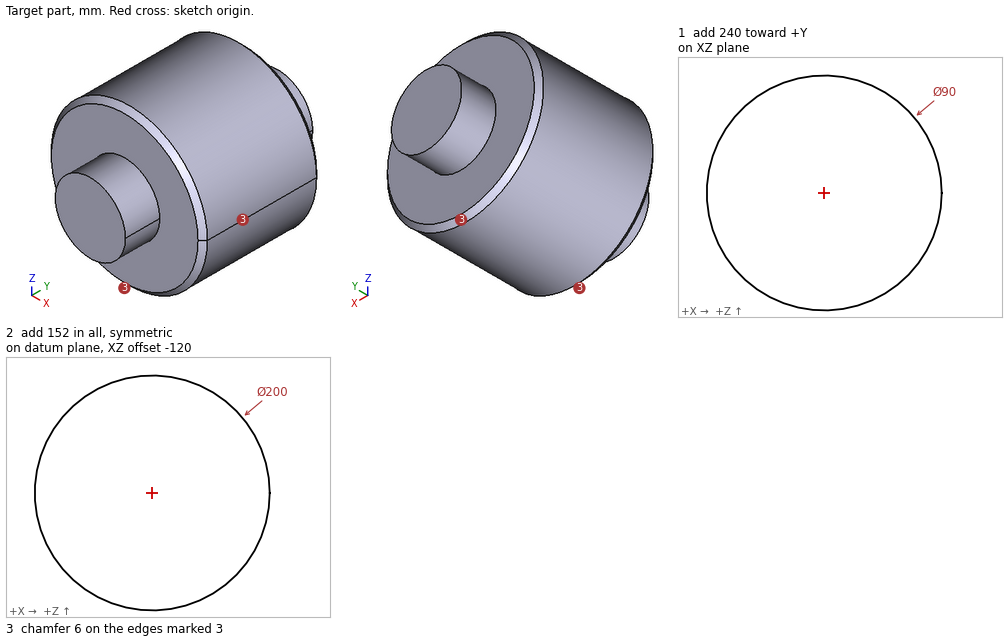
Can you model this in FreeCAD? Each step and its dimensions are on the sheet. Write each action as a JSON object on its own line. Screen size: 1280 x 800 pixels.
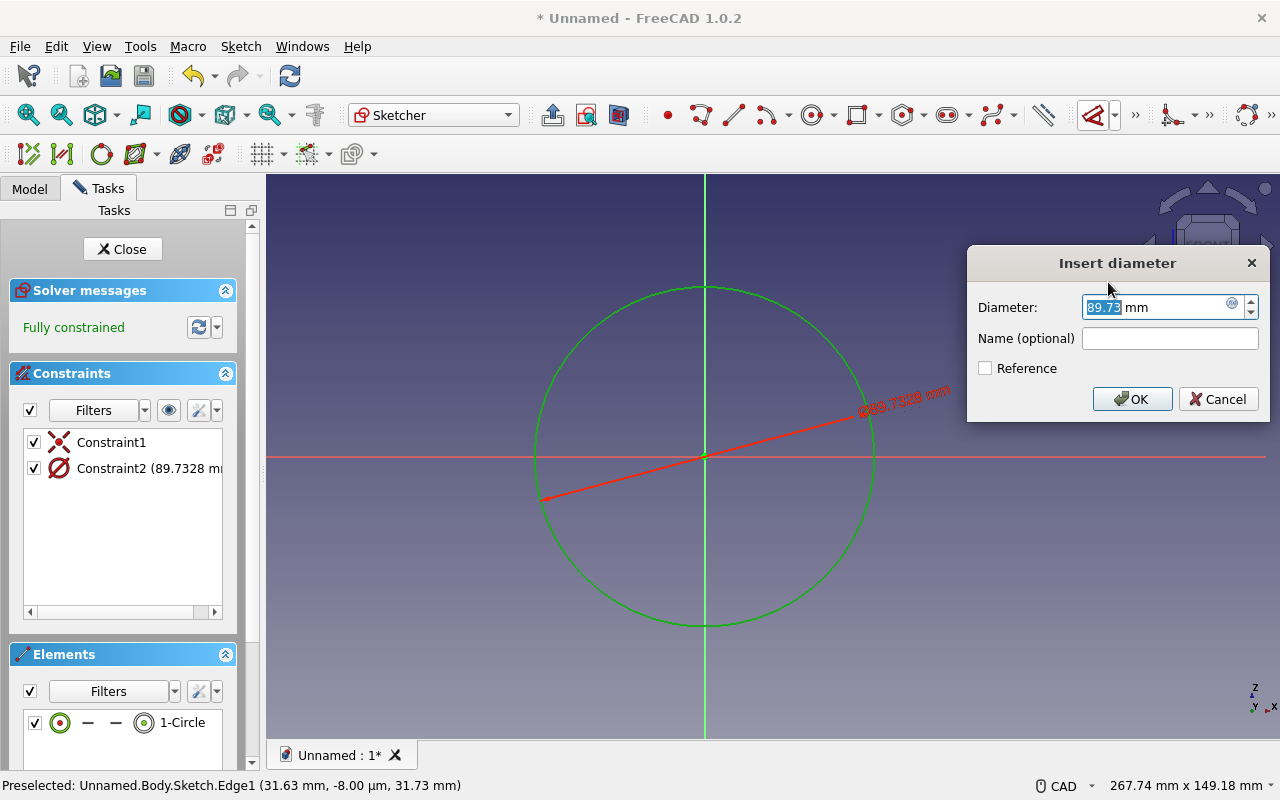
{"action": "type", "text": "90"}
{"action": "key", "text": "Return"}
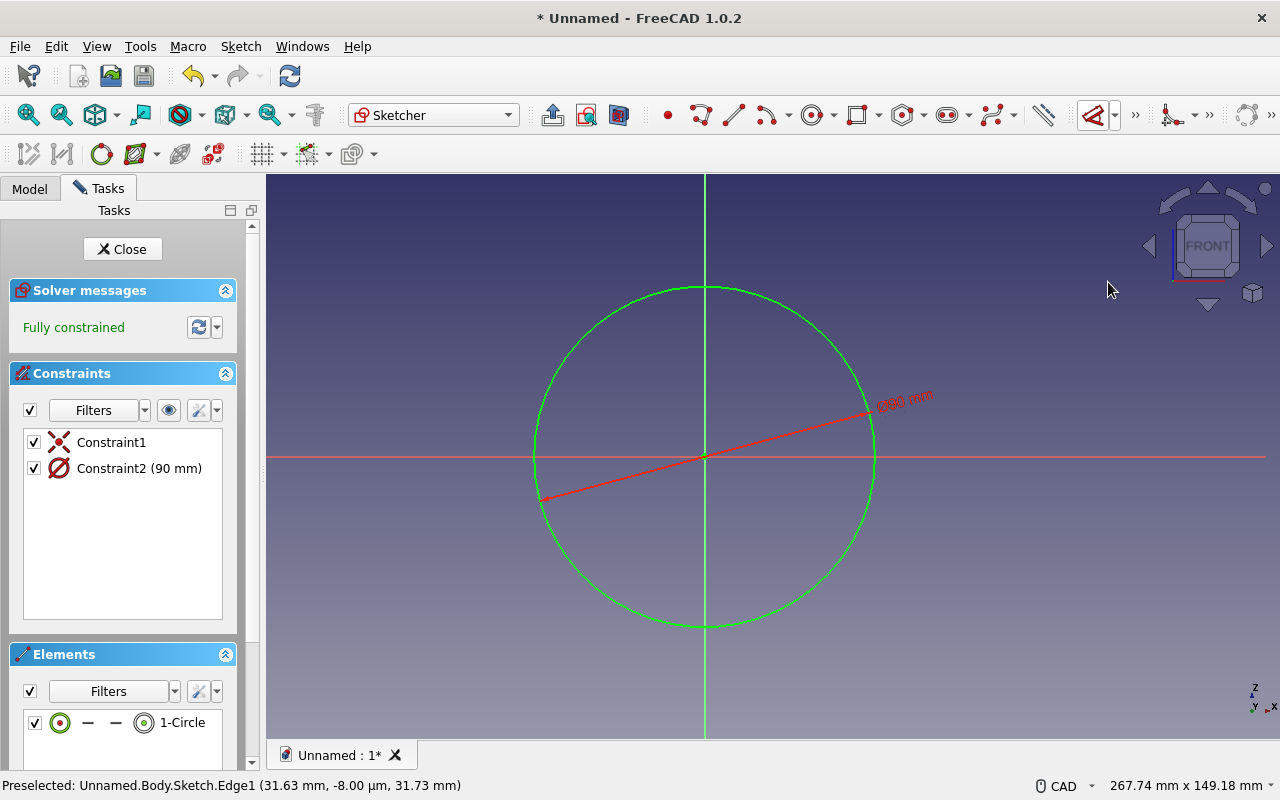
{"action": "left_click", "coordinate": [123, 249]}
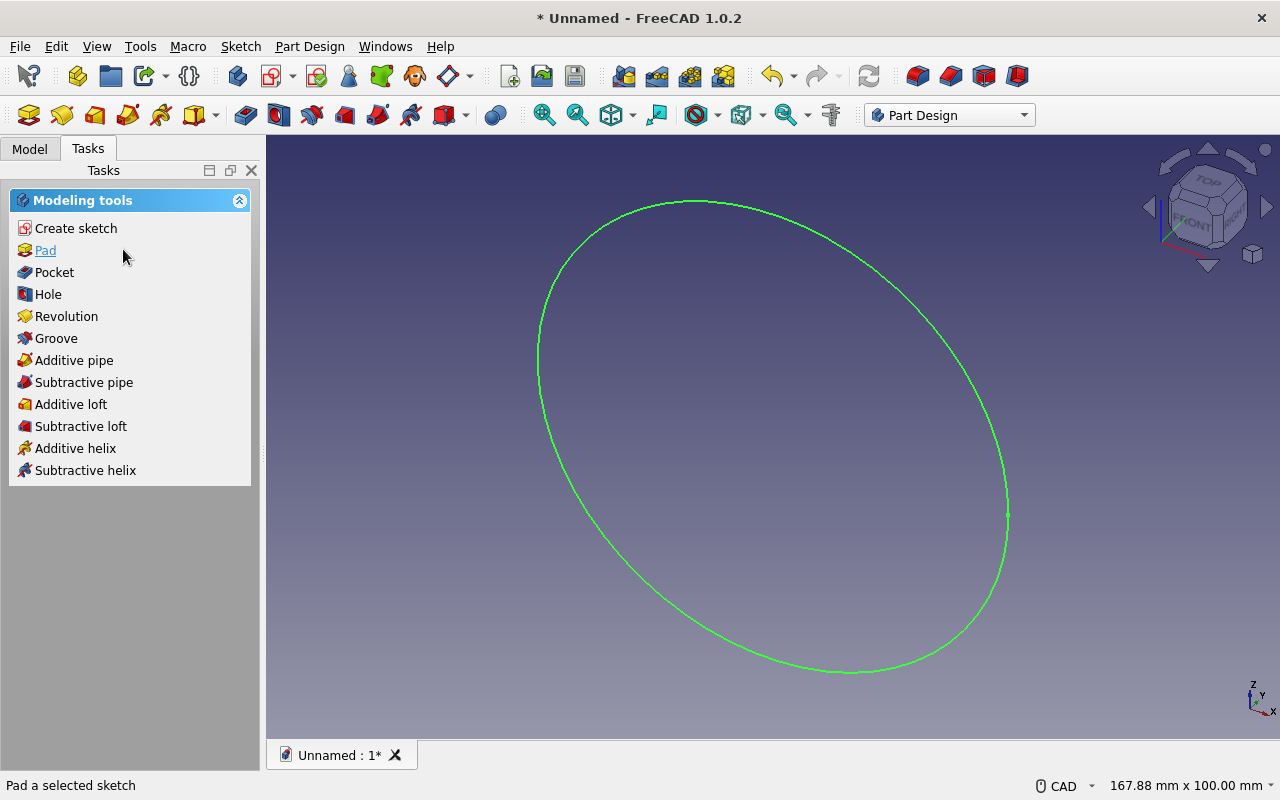
{"action": "left_click", "coordinate": [29, 116]}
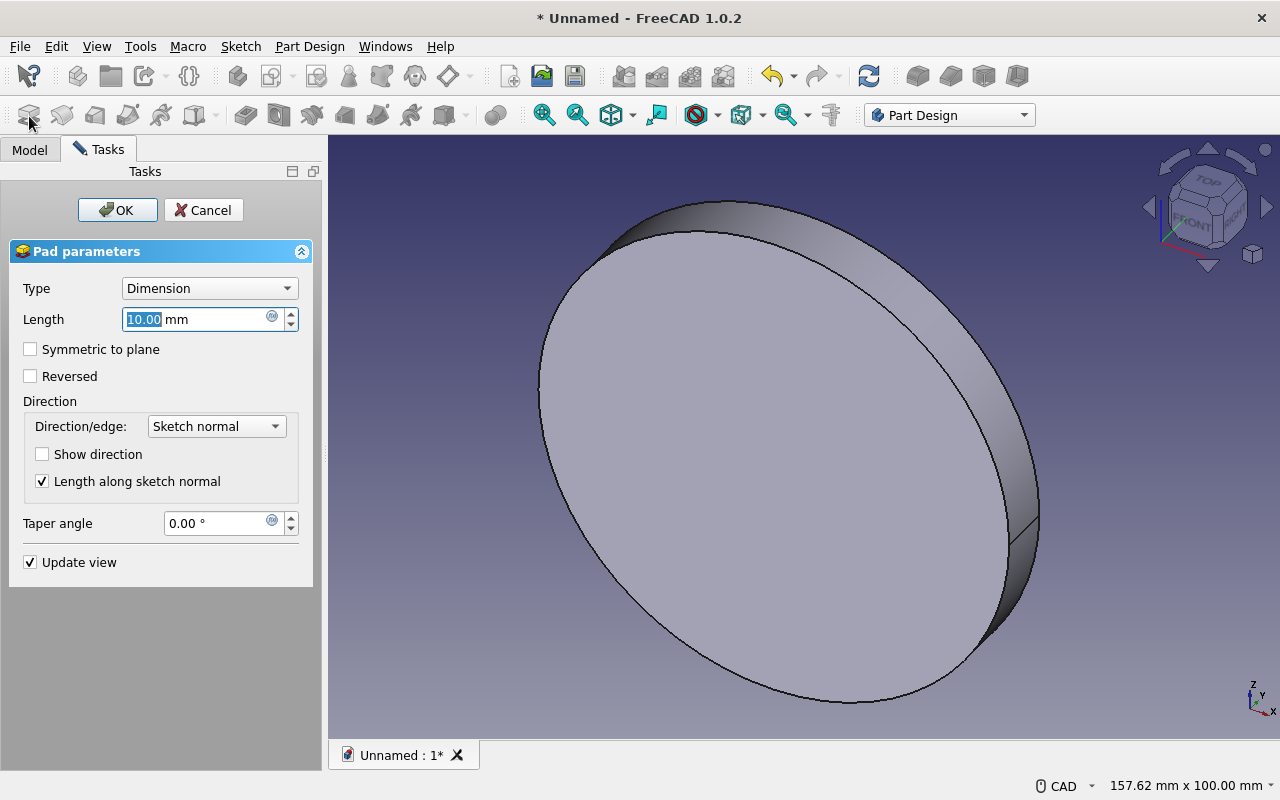
{"action": "type", "text": "240"}
{"action": "key", "text": "Tab"}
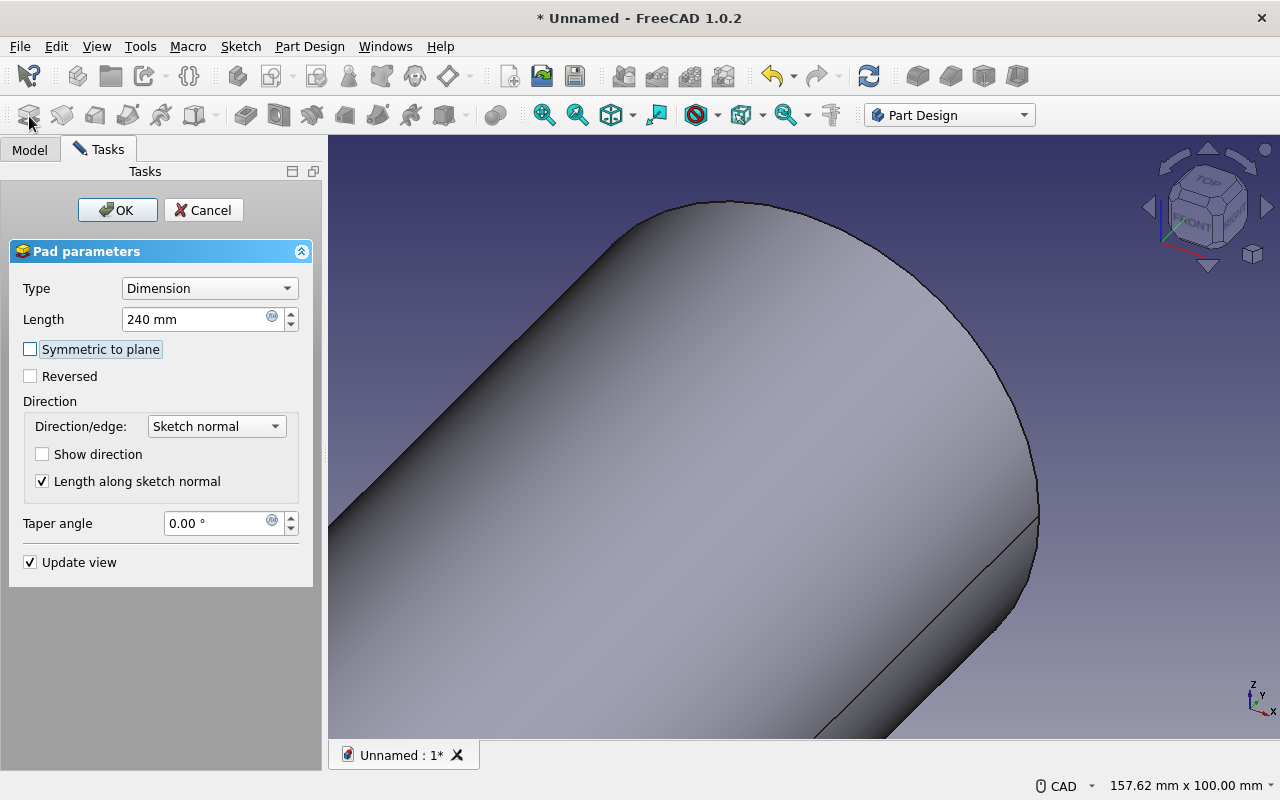
{"action": "left_click", "coordinate": [31, 376]}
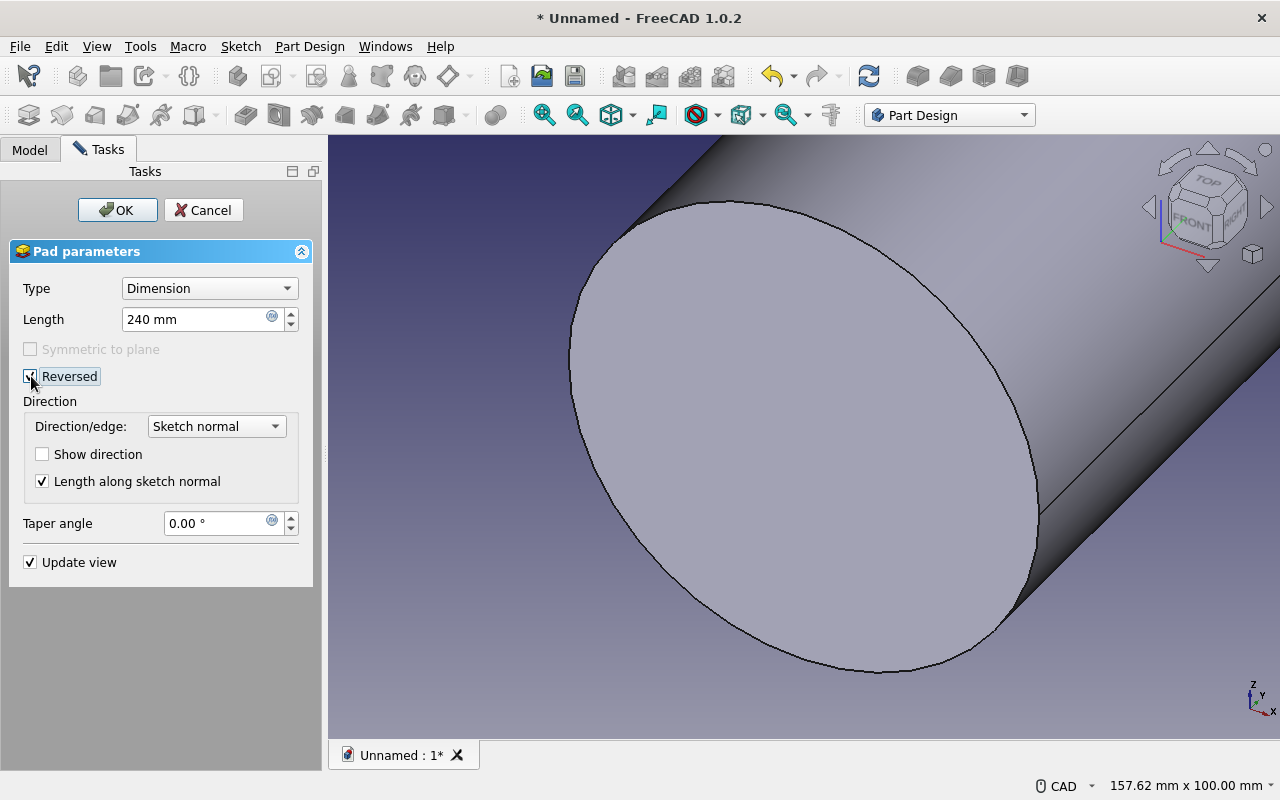
{"action": "left_click", "coordinate": [118, 210]}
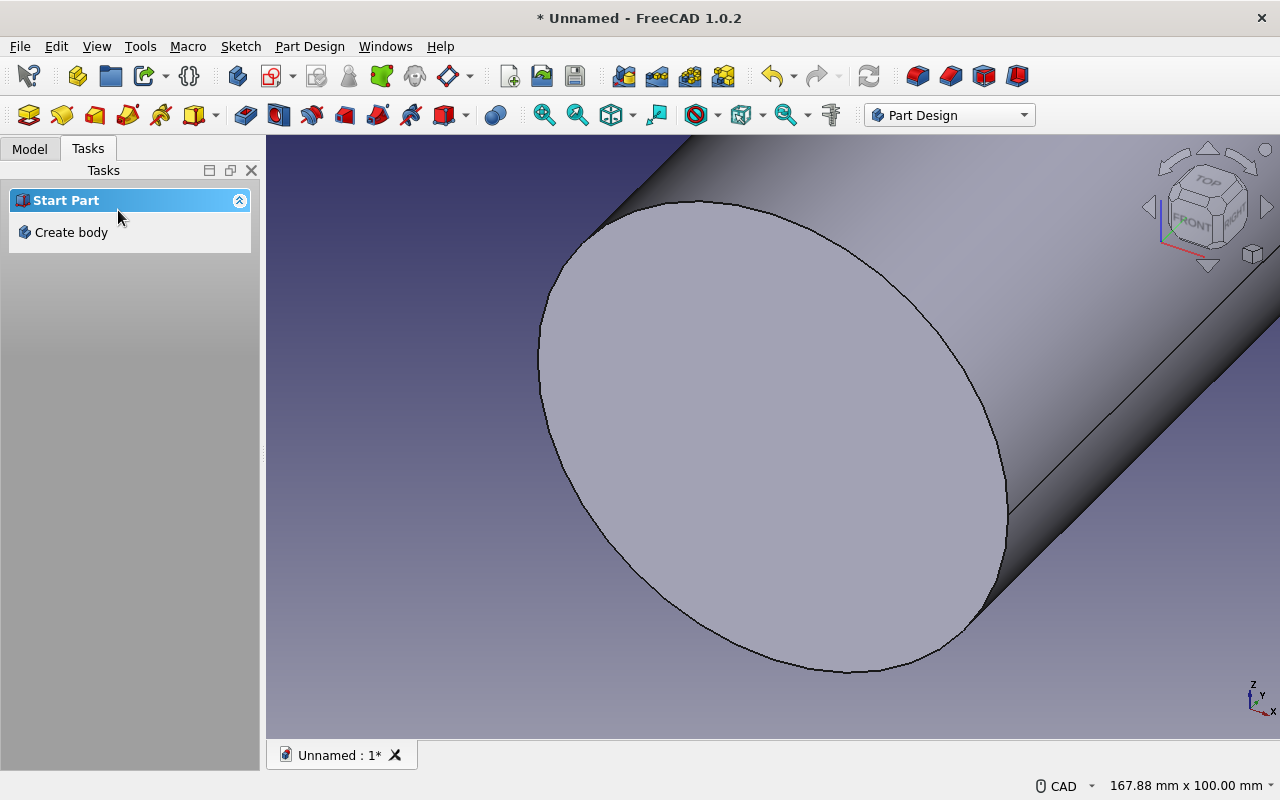
{"action": "left_click", "coordinate": [545, 116]}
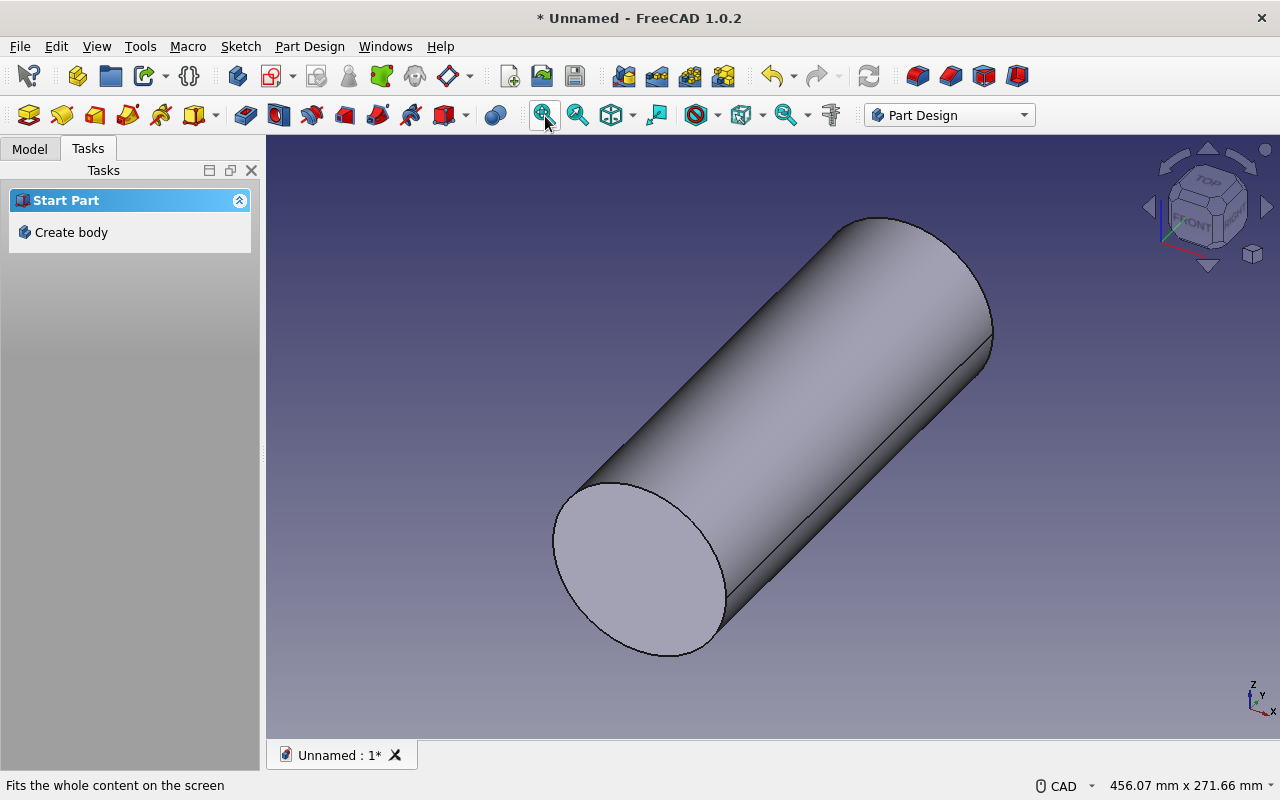
{"action": "left_click", "coordinate": [30, 148]}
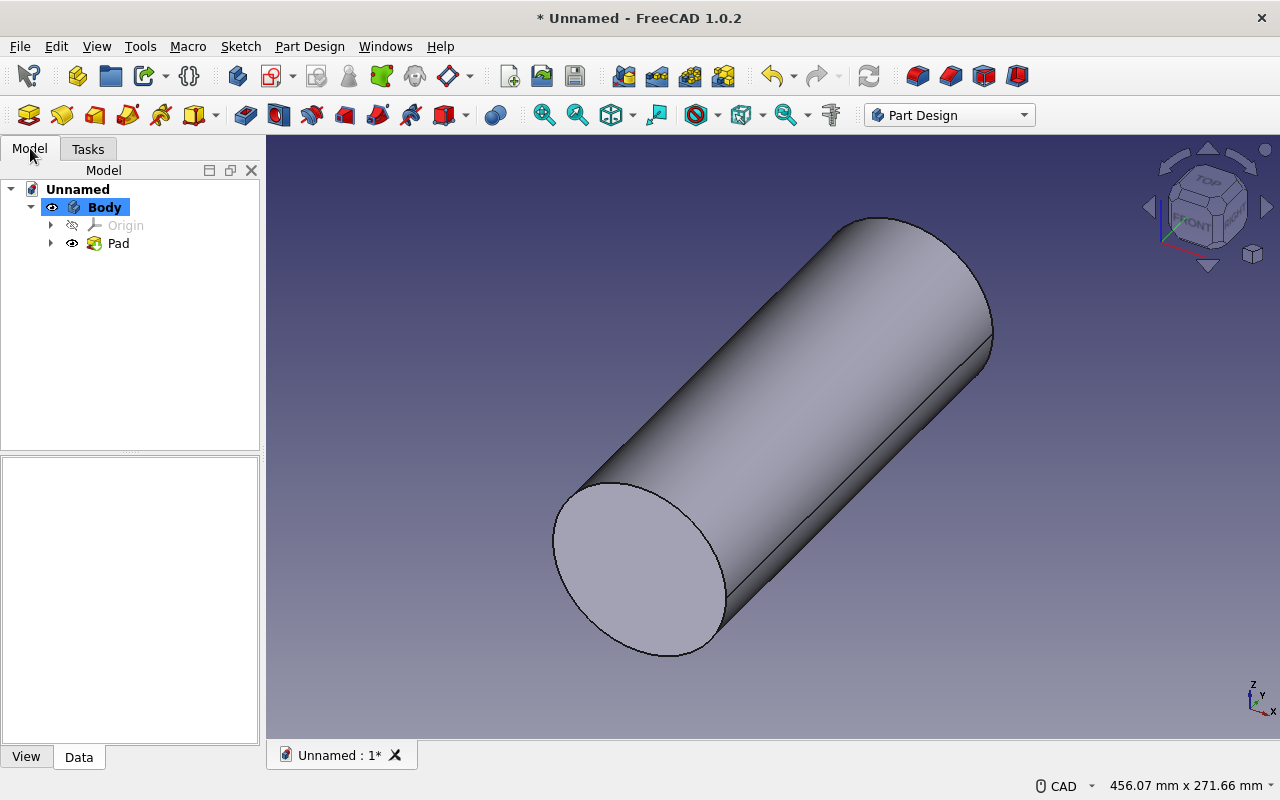
{"action": "left_click", "coordinate": [51, 225]}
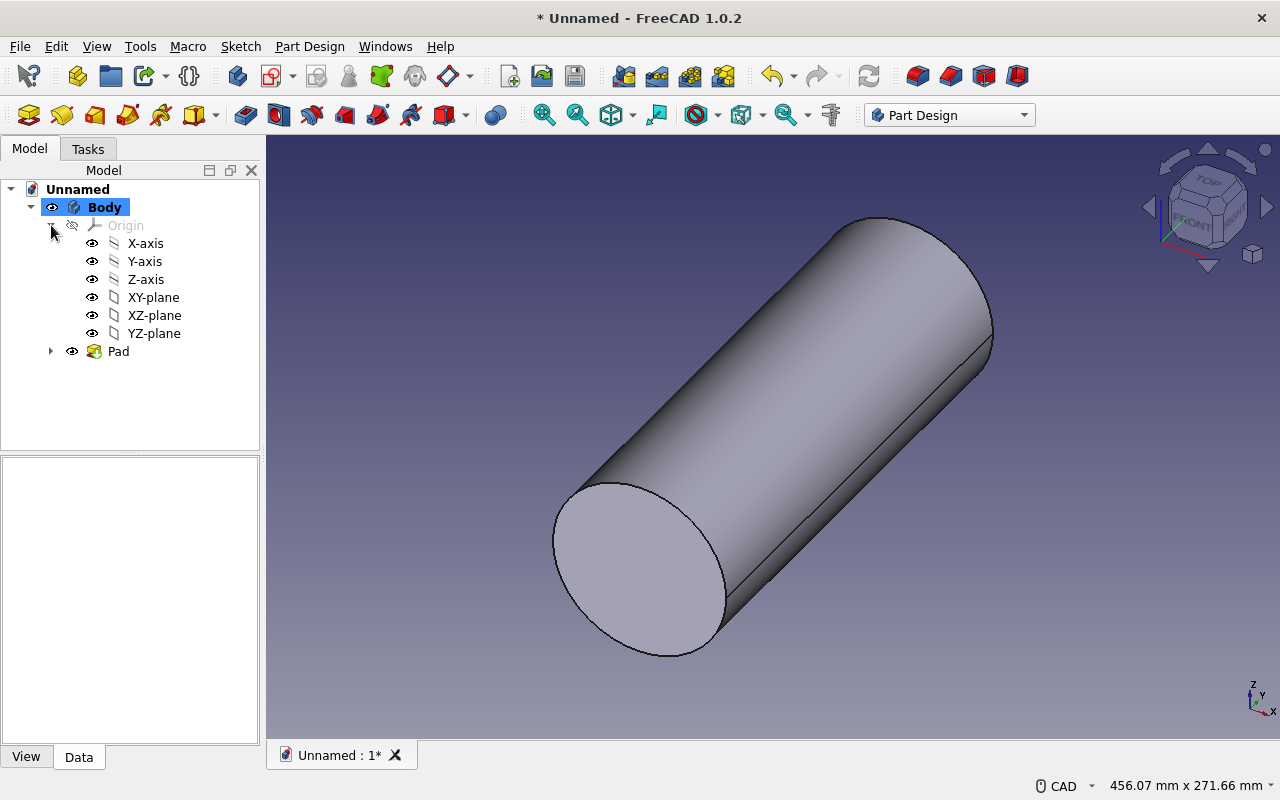
{"action": "left_click", "coordinate": [137, 315]}